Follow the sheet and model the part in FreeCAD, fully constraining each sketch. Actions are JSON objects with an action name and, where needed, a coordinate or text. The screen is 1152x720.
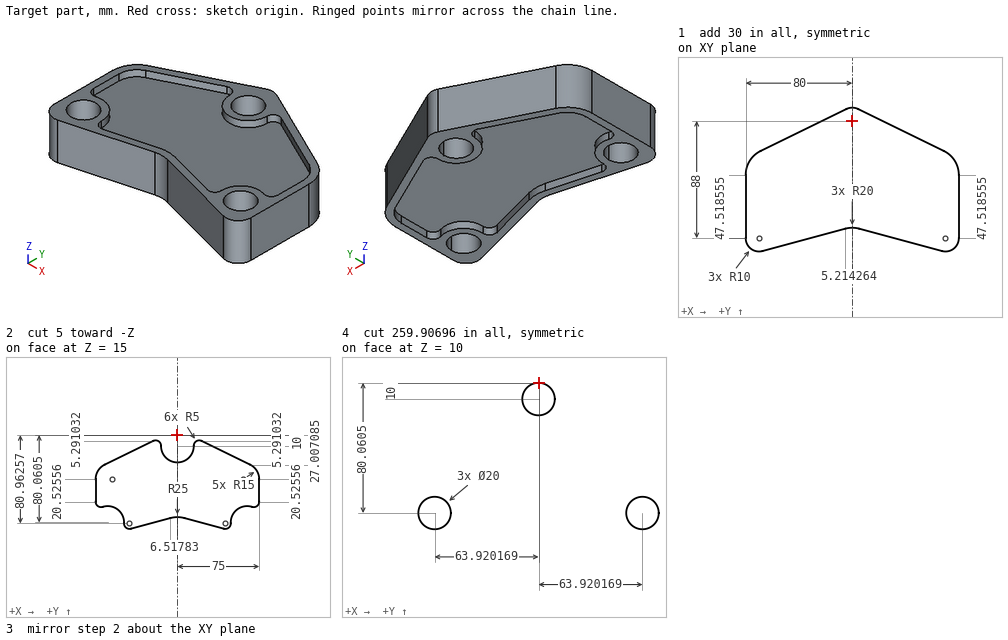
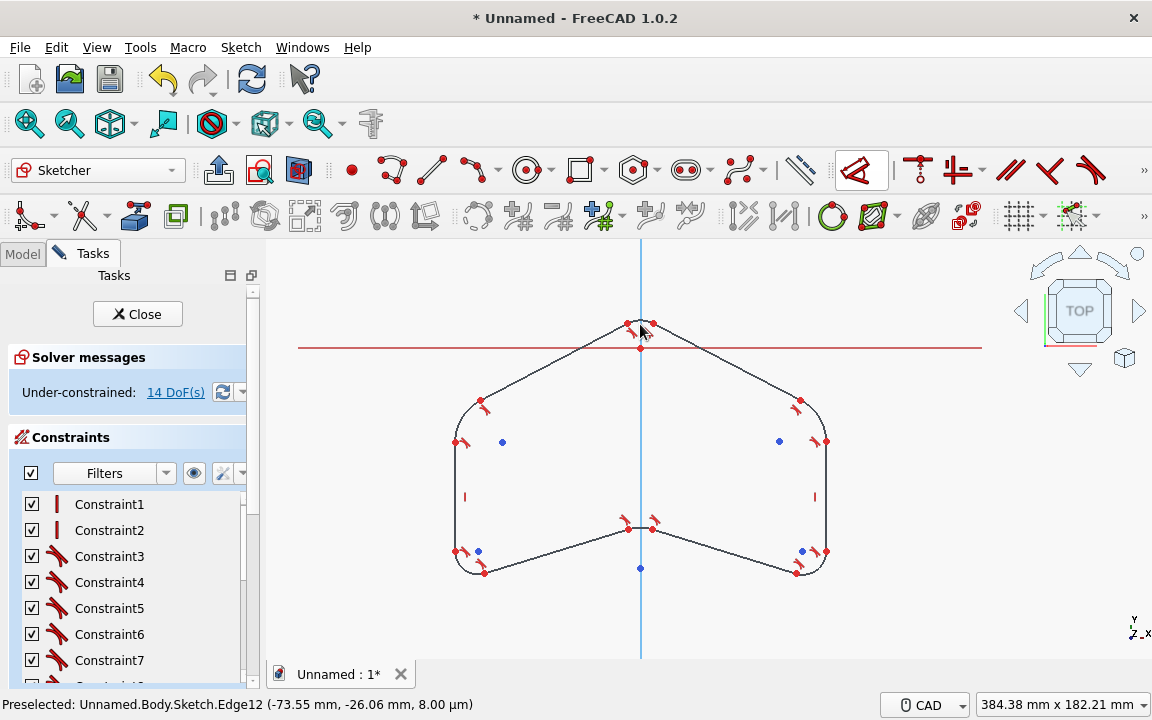
{"action": "left_click", "coordinate": [459, 564]}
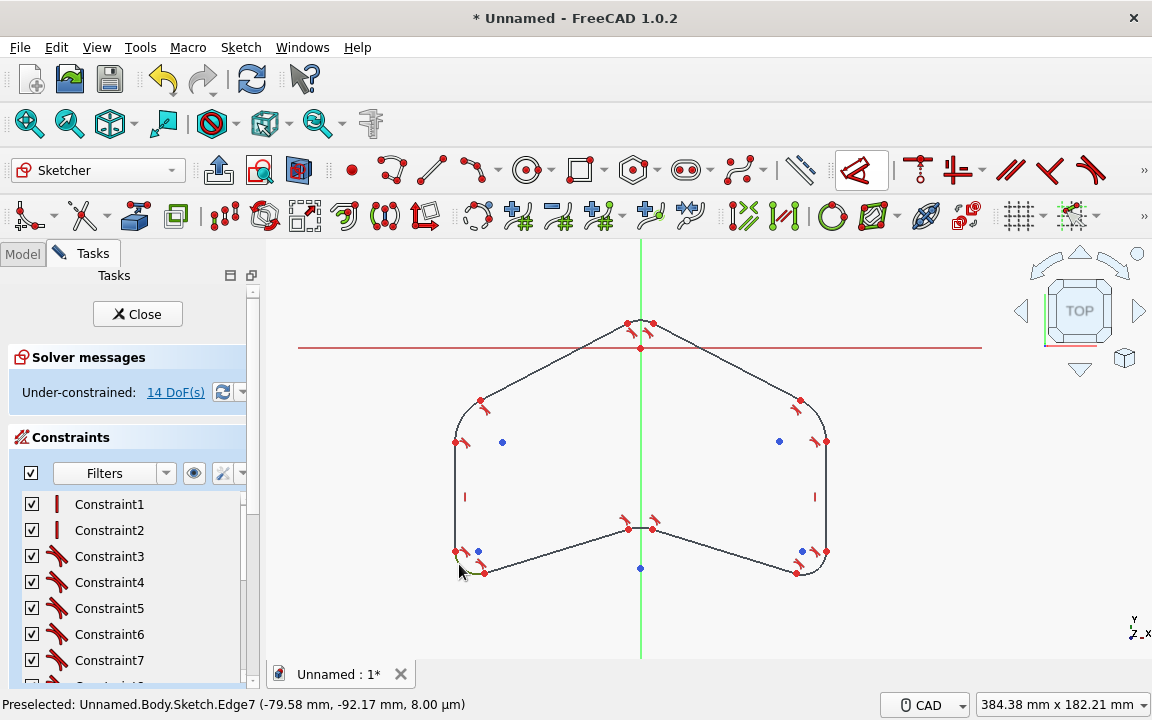
{"action": "left_click", "coordinate": [809, 574]}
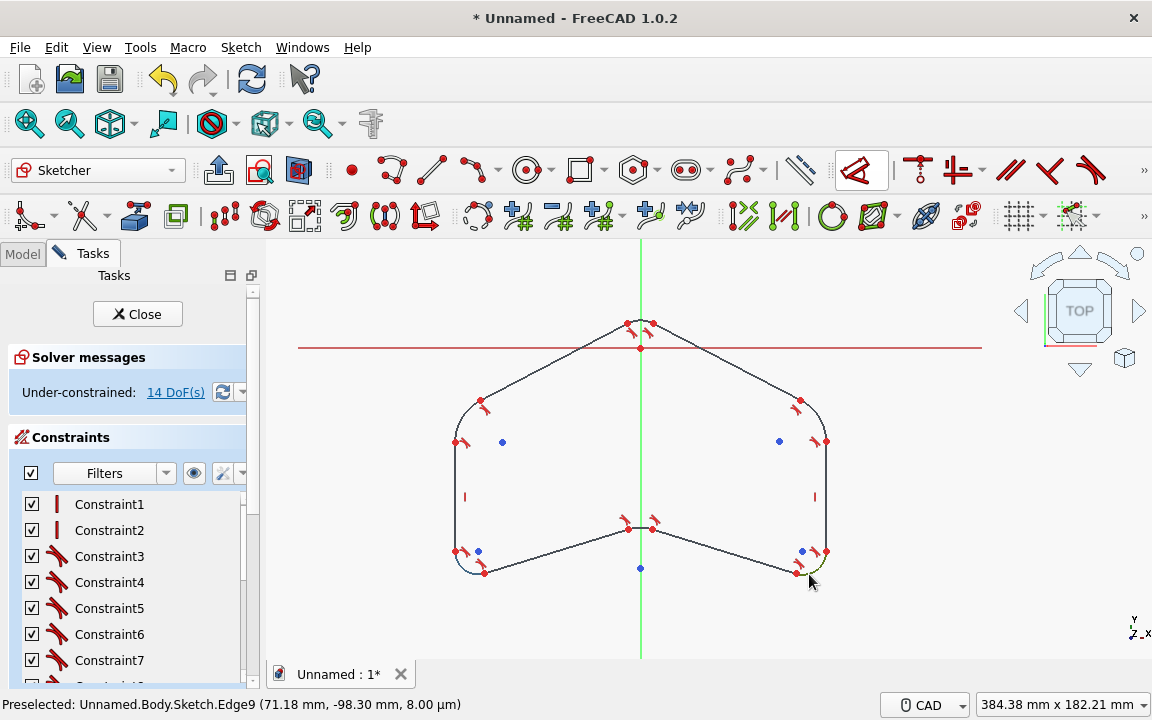
{"action": "left_click", "coordinate": [641, 320]}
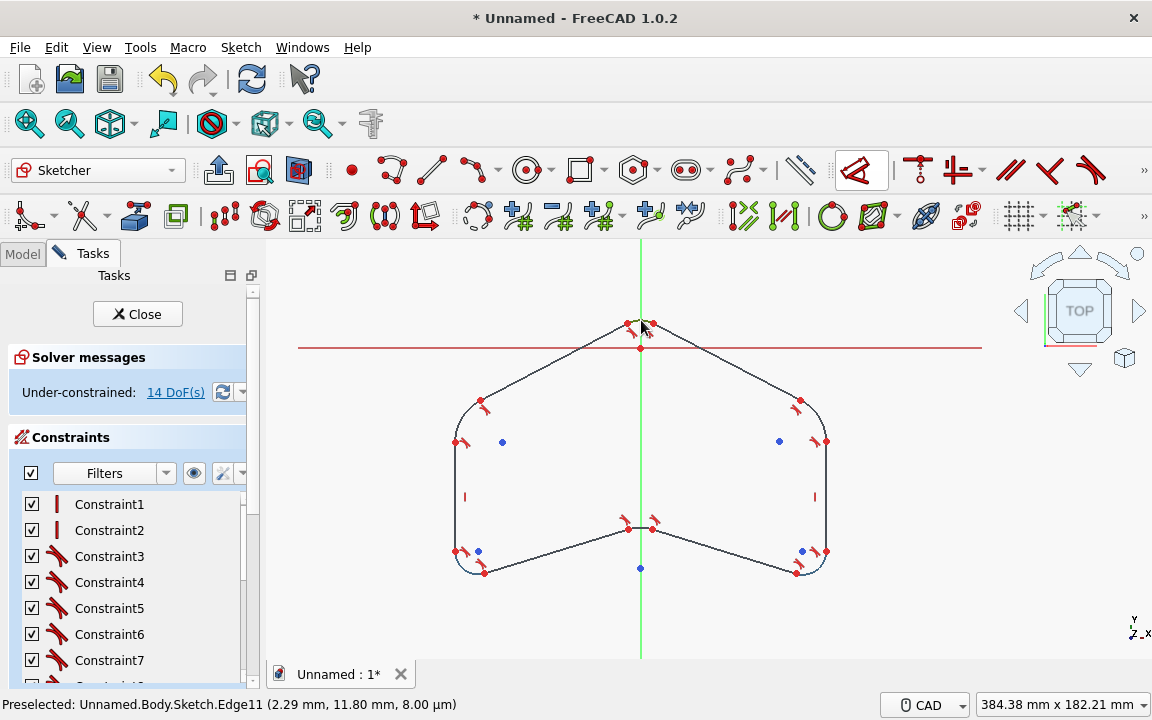
{"action": "key", "text": "e"}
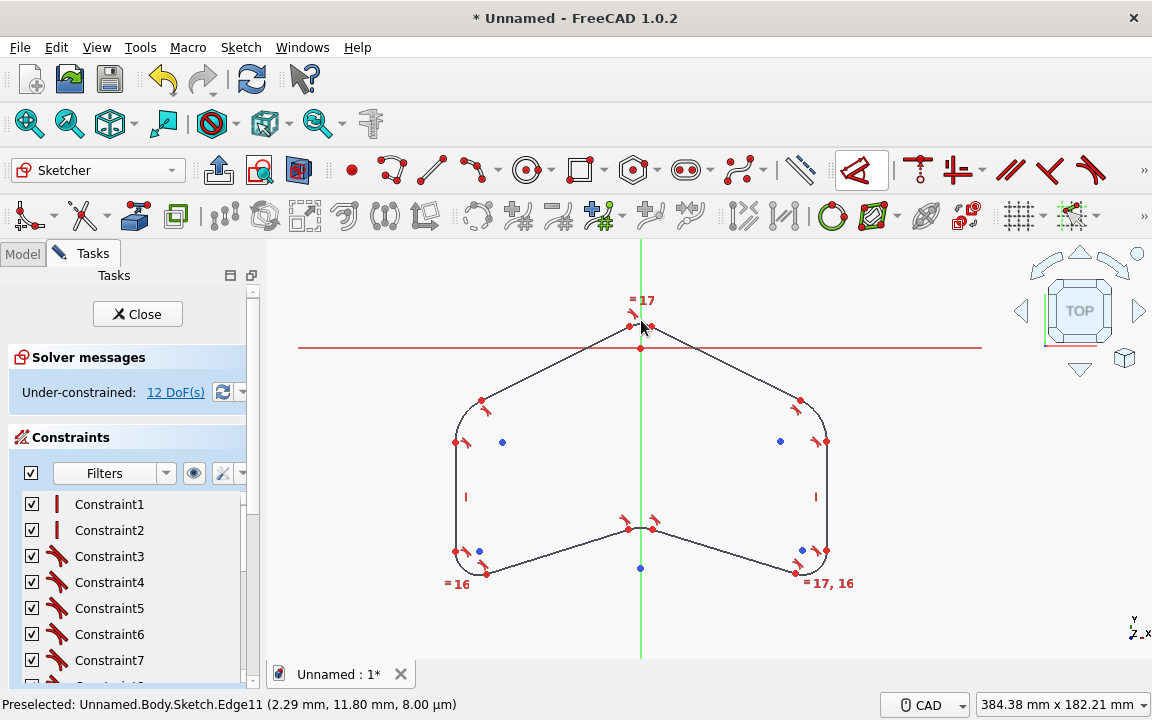
{"action": "left_click", "coordinate": [640, 528]}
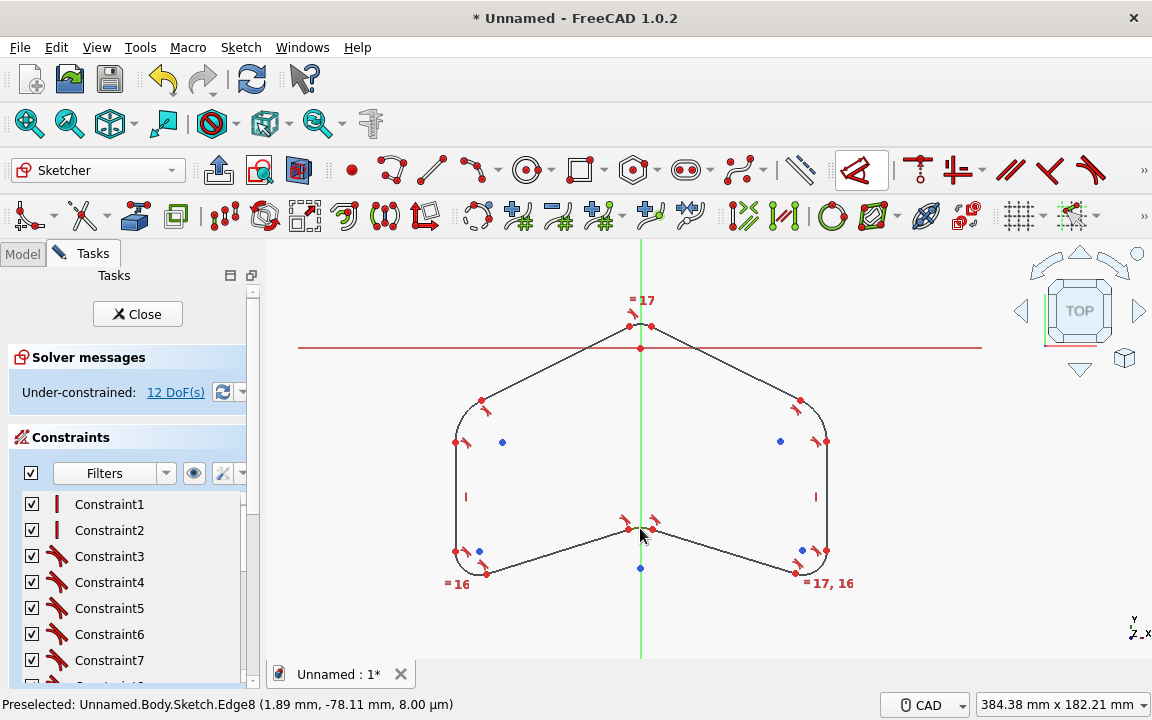
{"action": "left_click", "coordinate": [824, 427]}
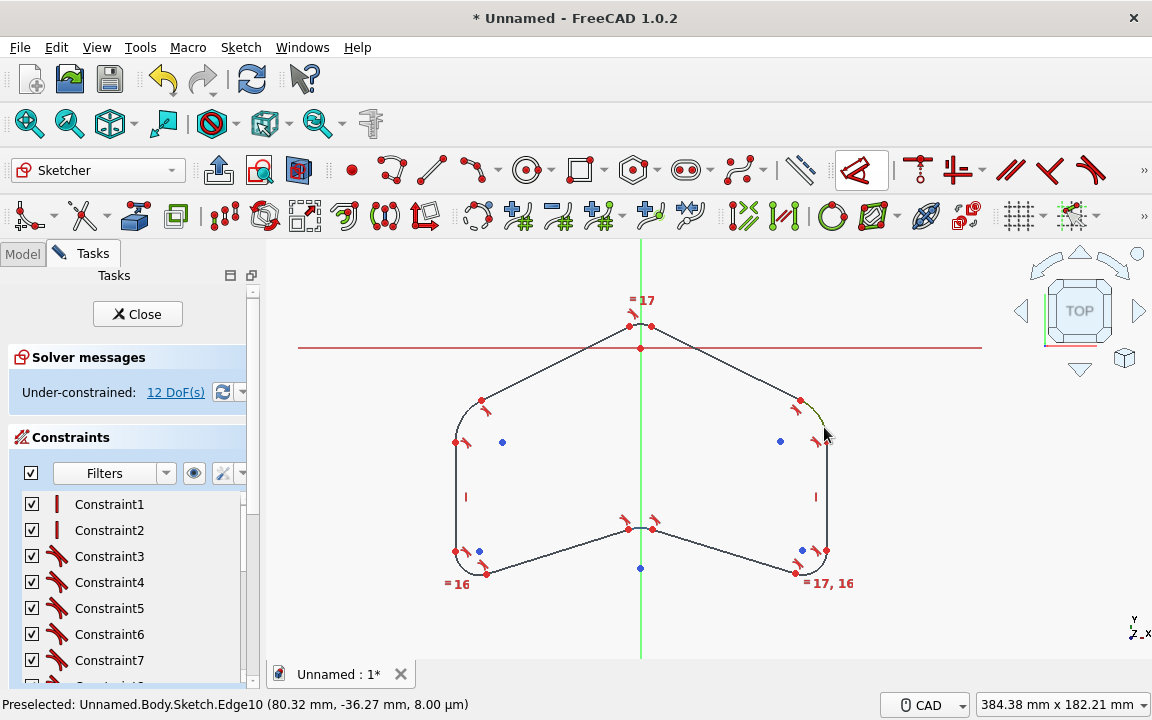
{"action": "left_click", "coordinate": [469, 410]}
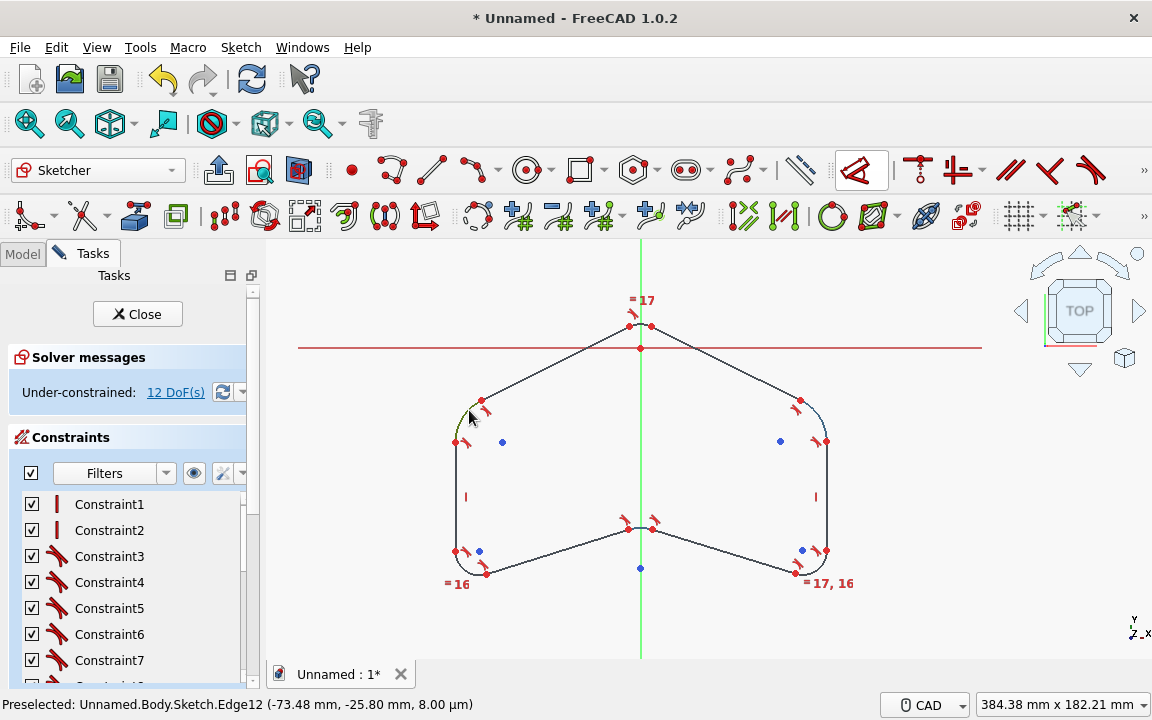
{"action": "key", "text": "e"}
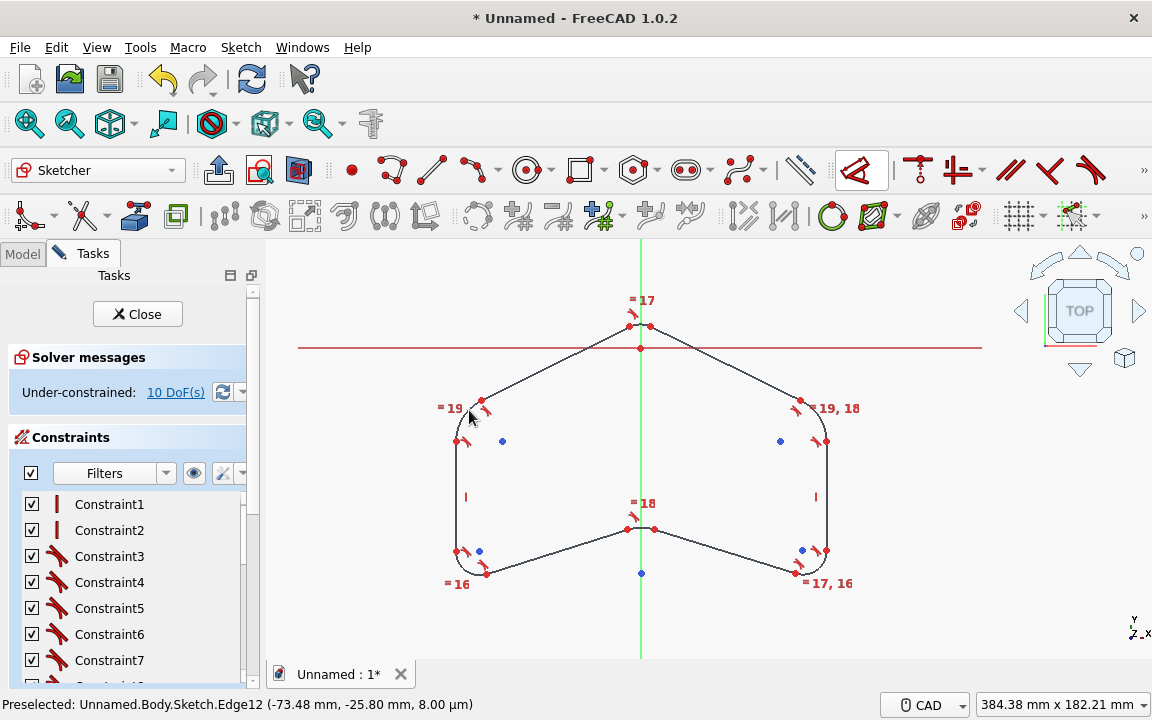
{"action": "left_click", "coordinate": [641, 574]}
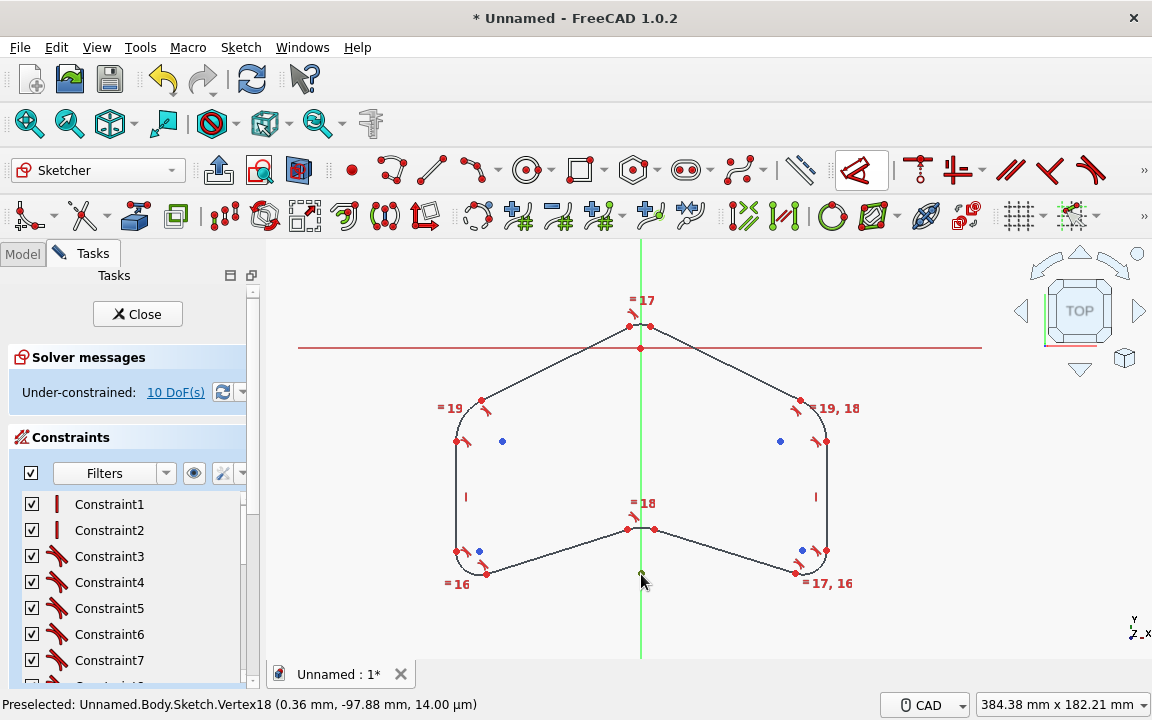
{"action": "left_click", "coordinate": [641, 605]}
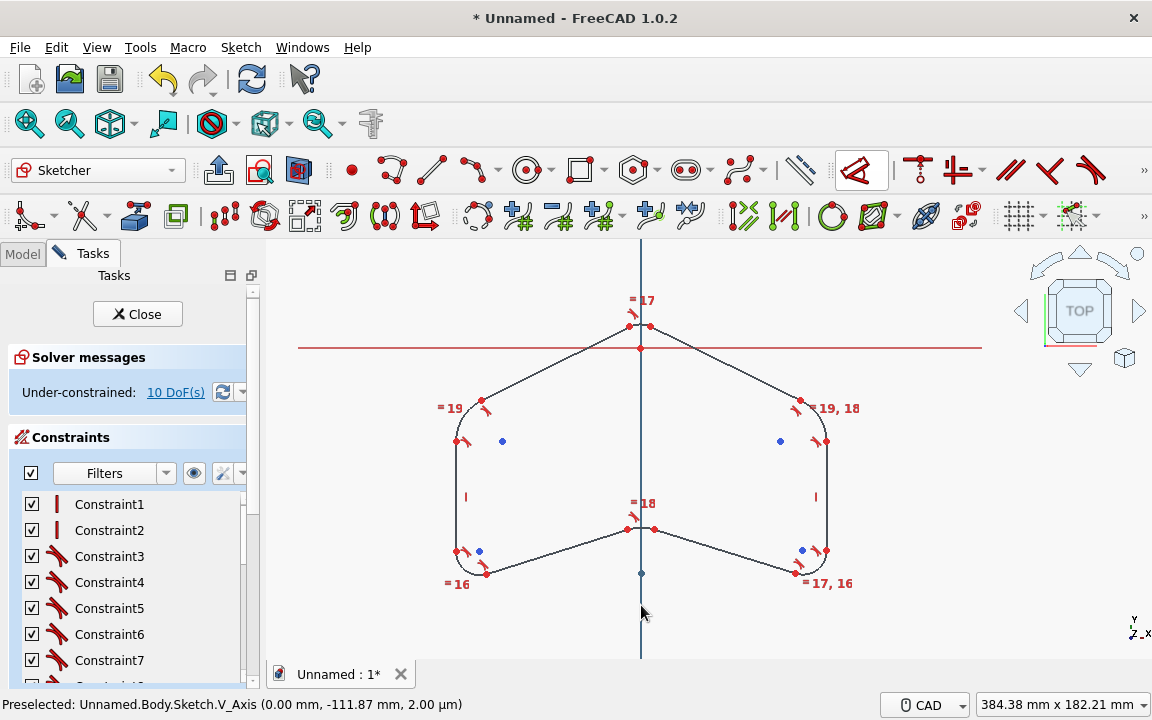
{"action": "left_click", "coordinate": [918, 170]}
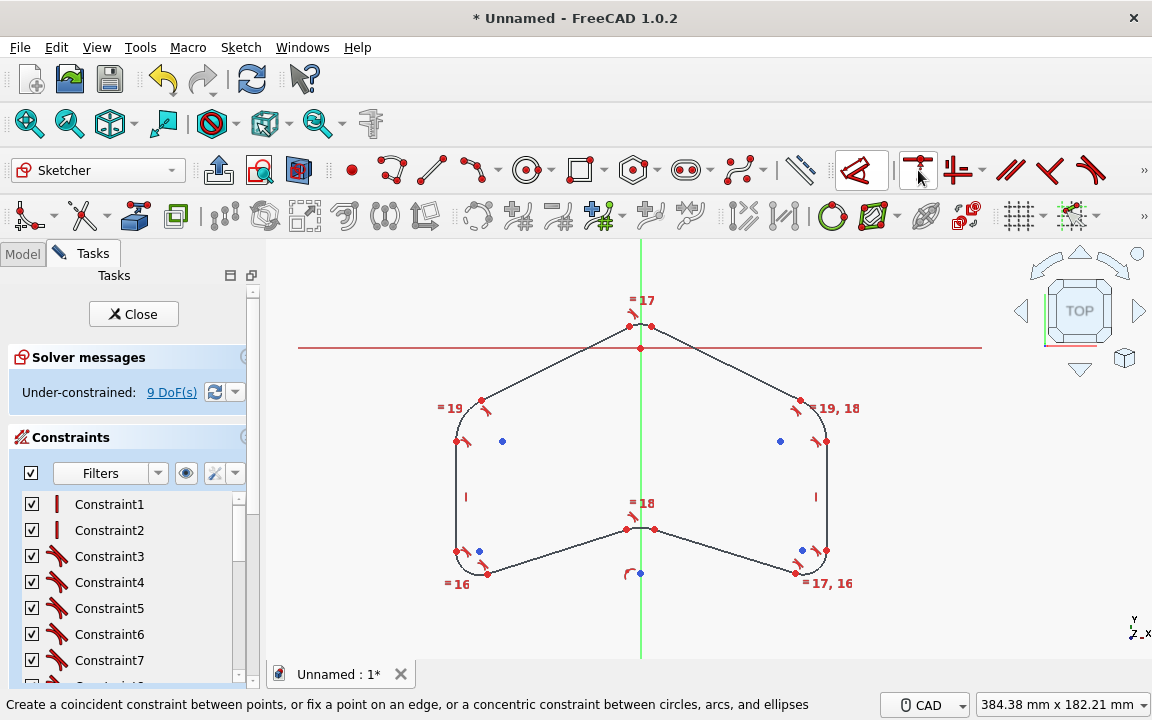
{"action": "left_click", "coordinate": [480, 552]}